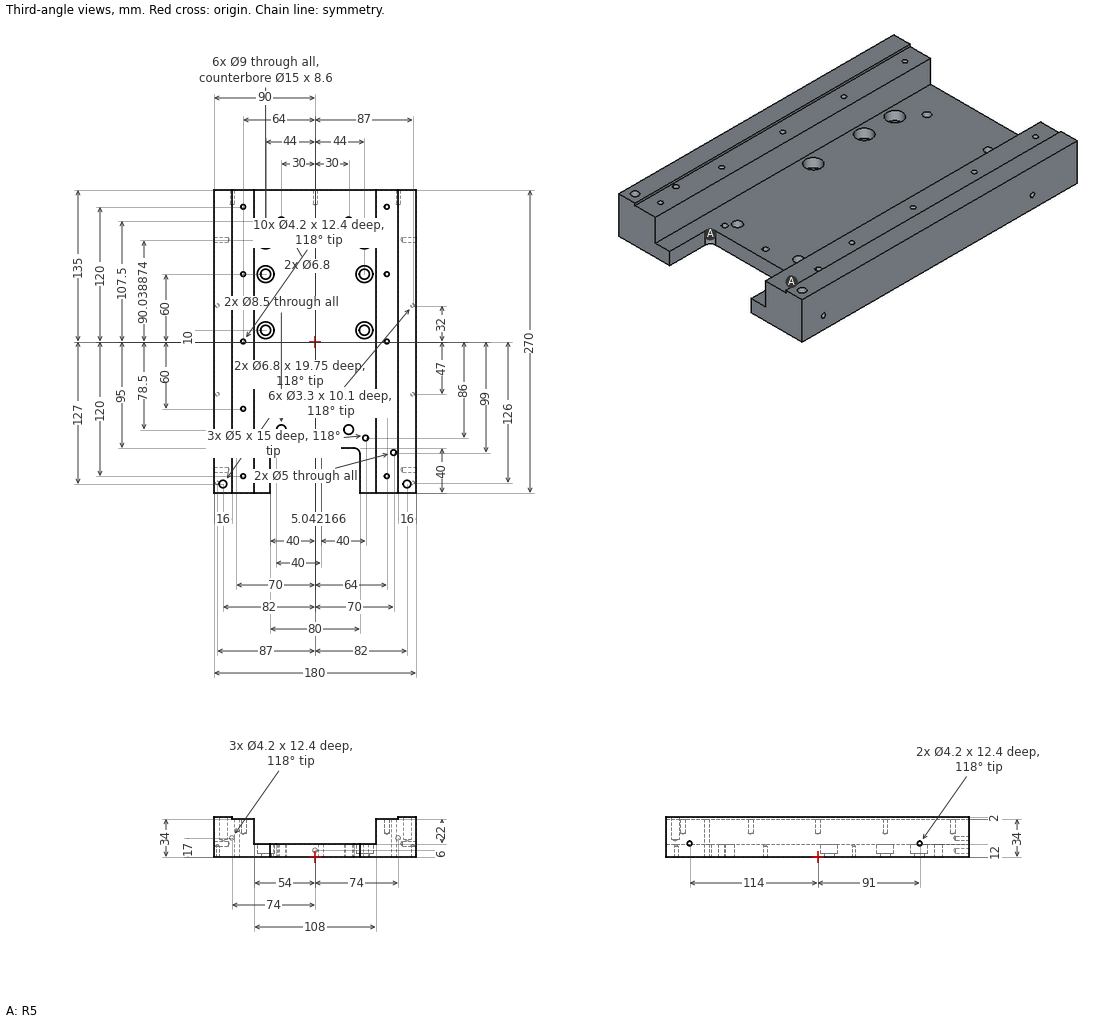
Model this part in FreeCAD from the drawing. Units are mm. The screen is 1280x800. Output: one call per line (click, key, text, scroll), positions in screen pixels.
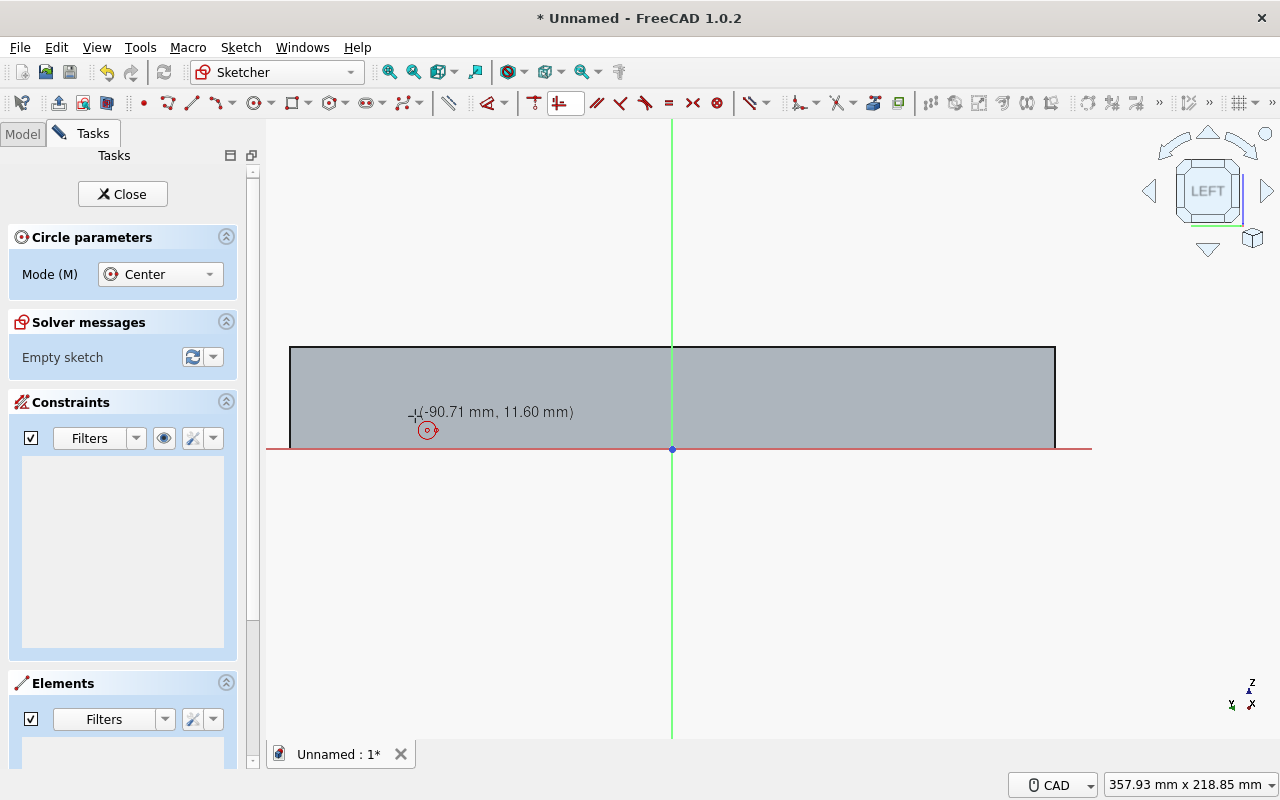
click(414, 415)
move(419, 411)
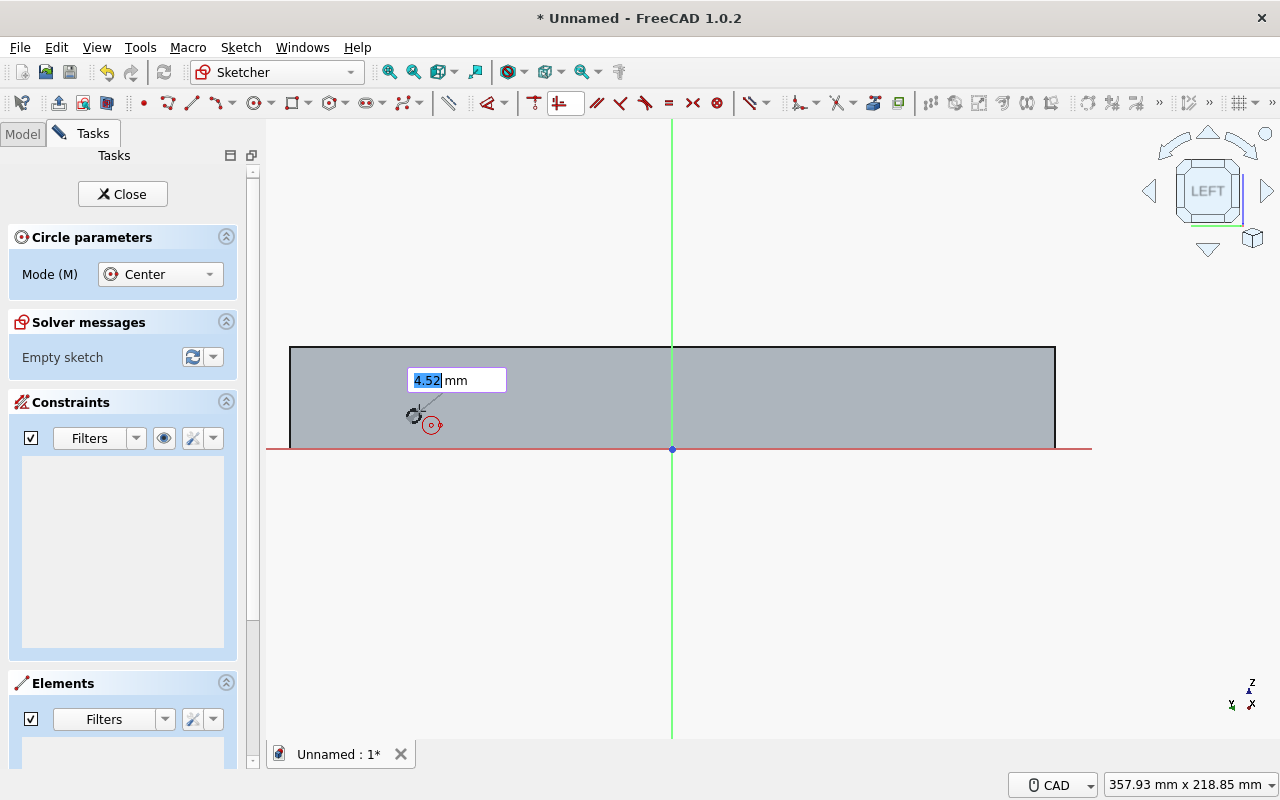
text(4.2)
key(Return)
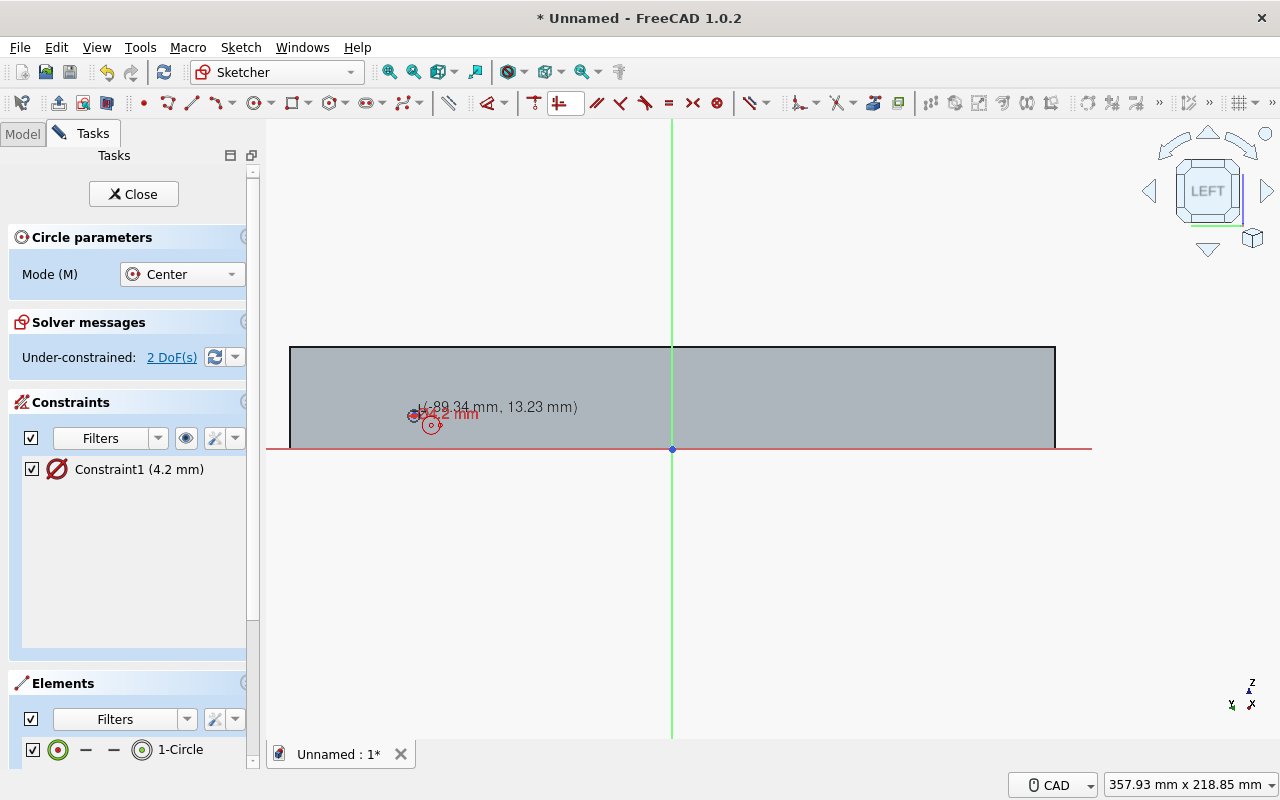
scroll(995, 415, up, 7)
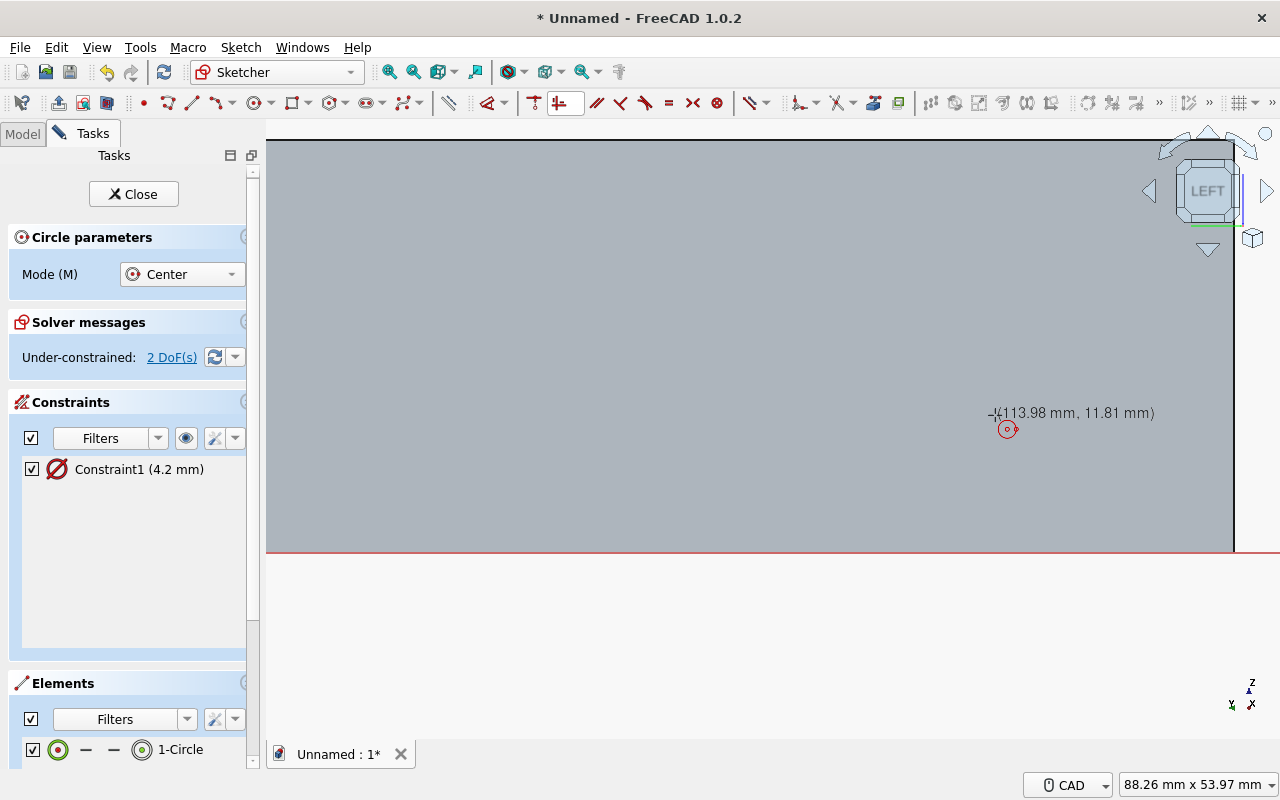
scroll(995, 415, down, 7)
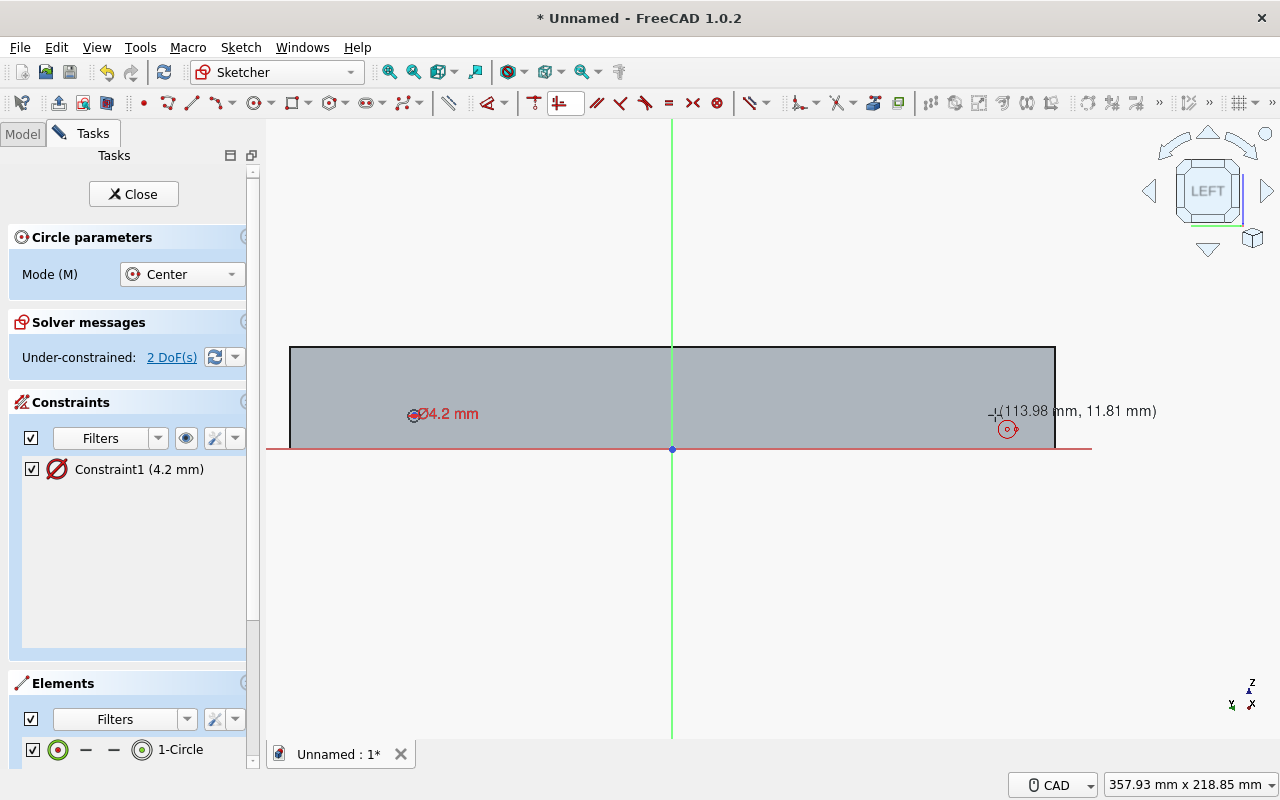
click(995, 415)
move(999, 411)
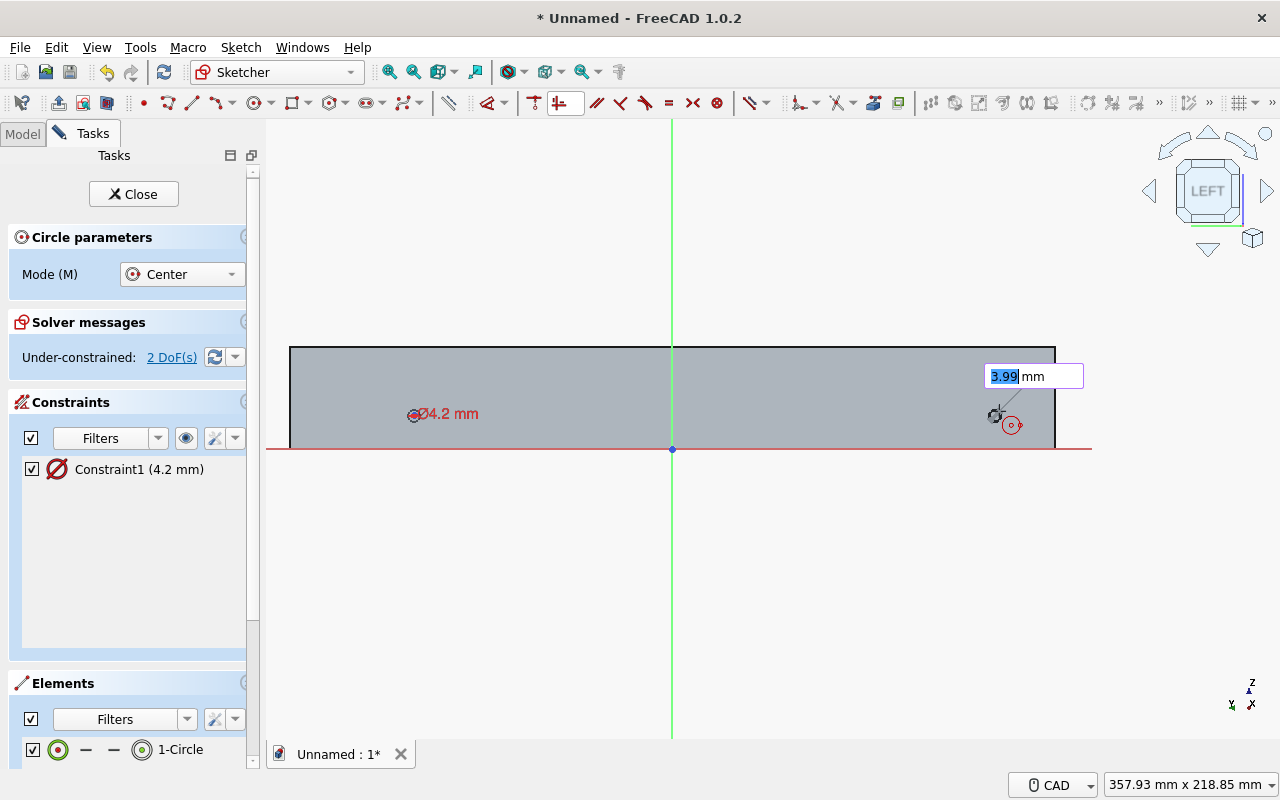
text(4.2)
key(Return)
key(Escape)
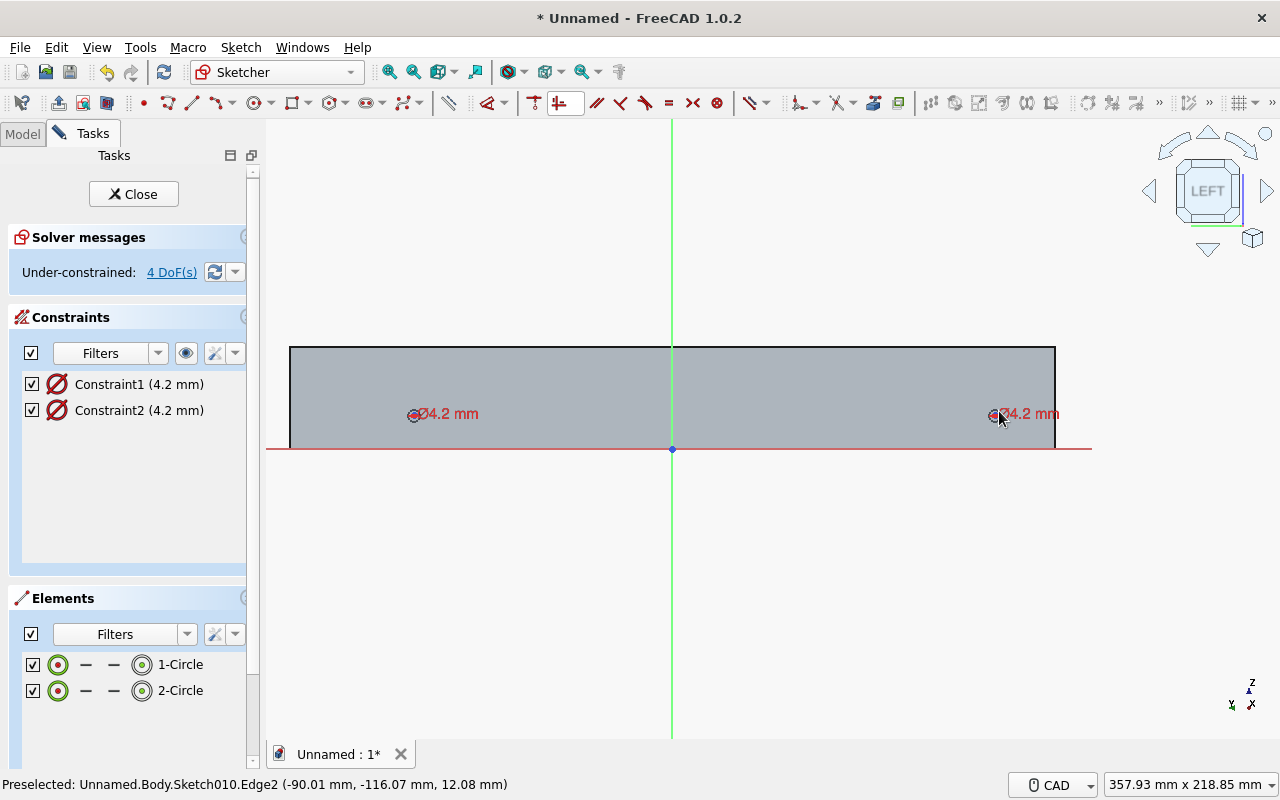
click(414, 416)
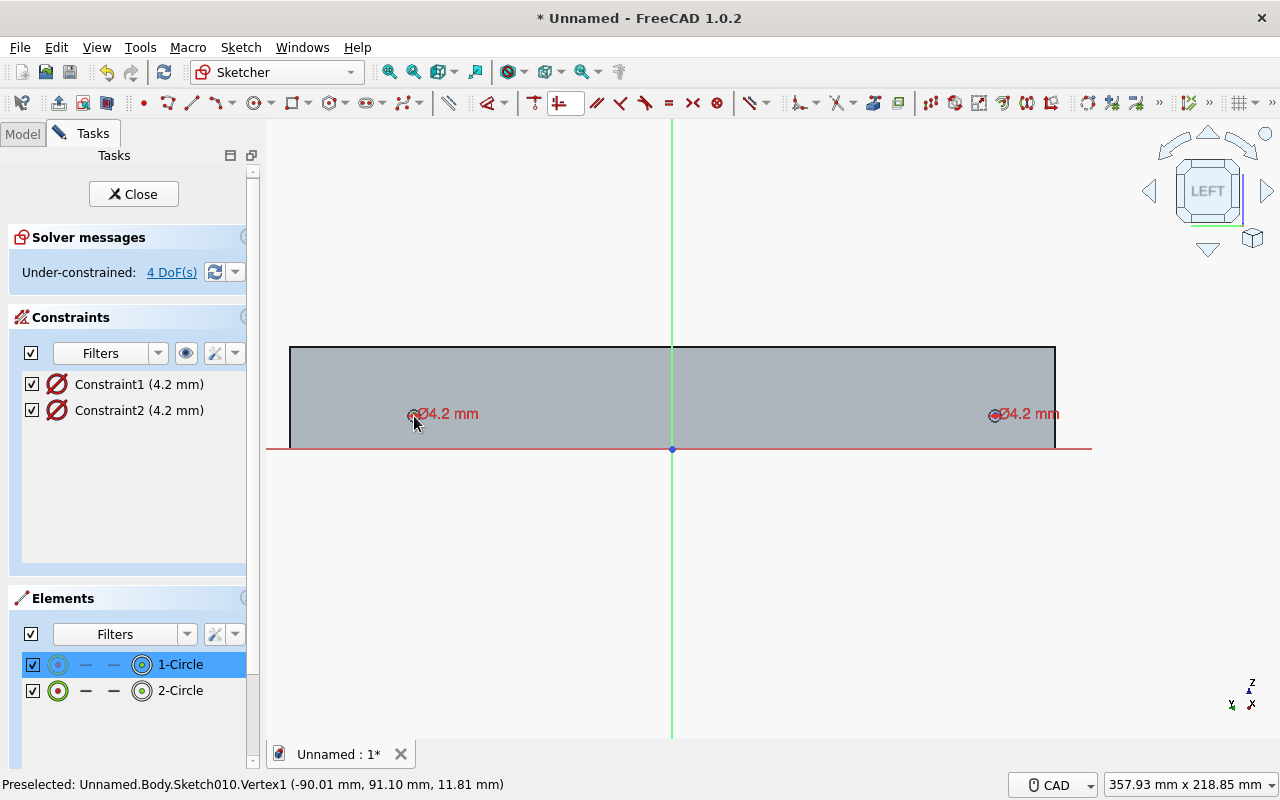
click(995, 416)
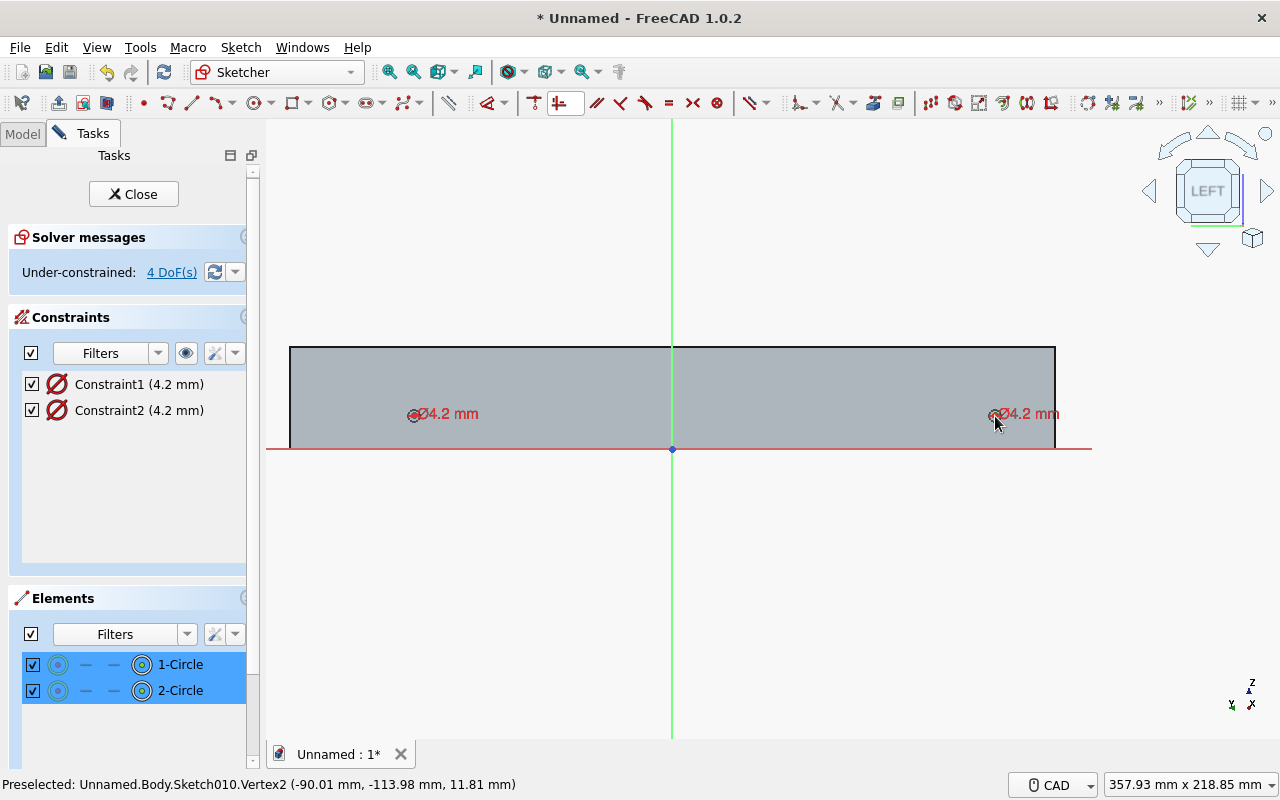
click(578, 104)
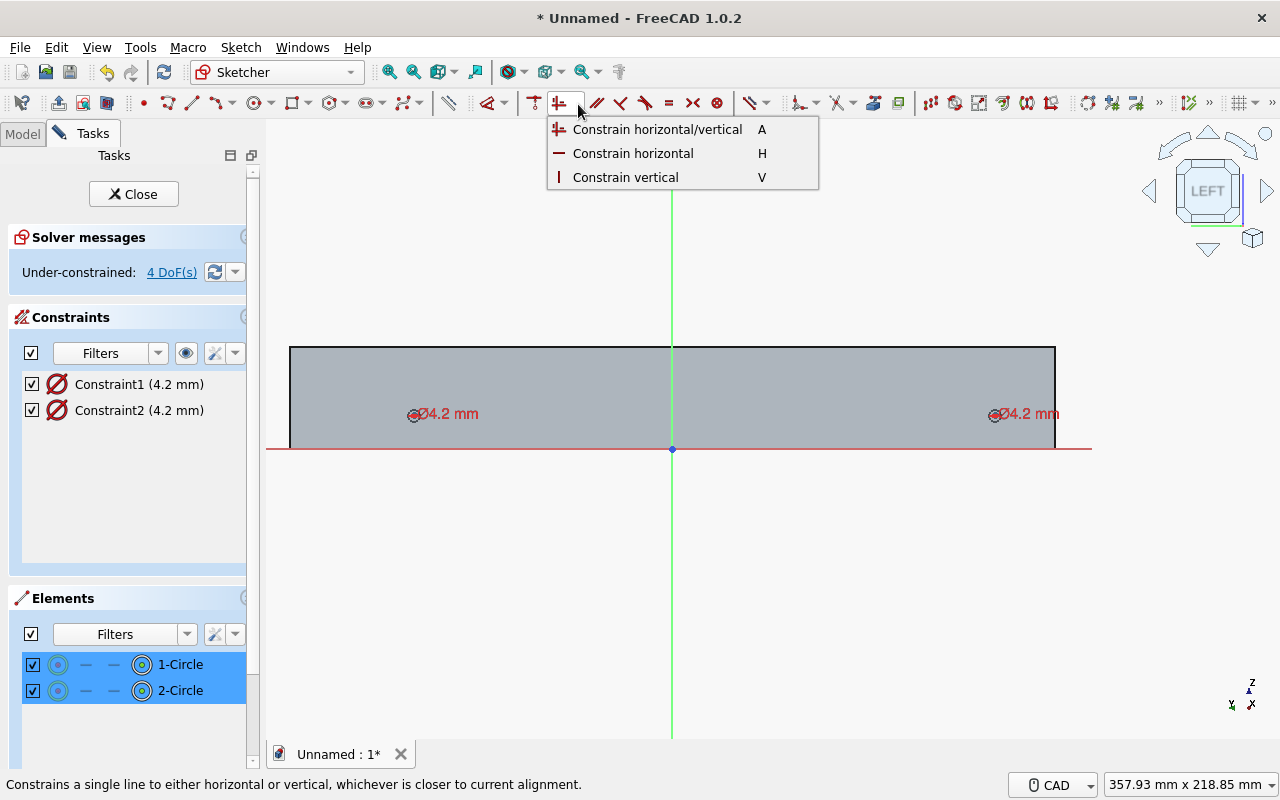
click(683, 153)